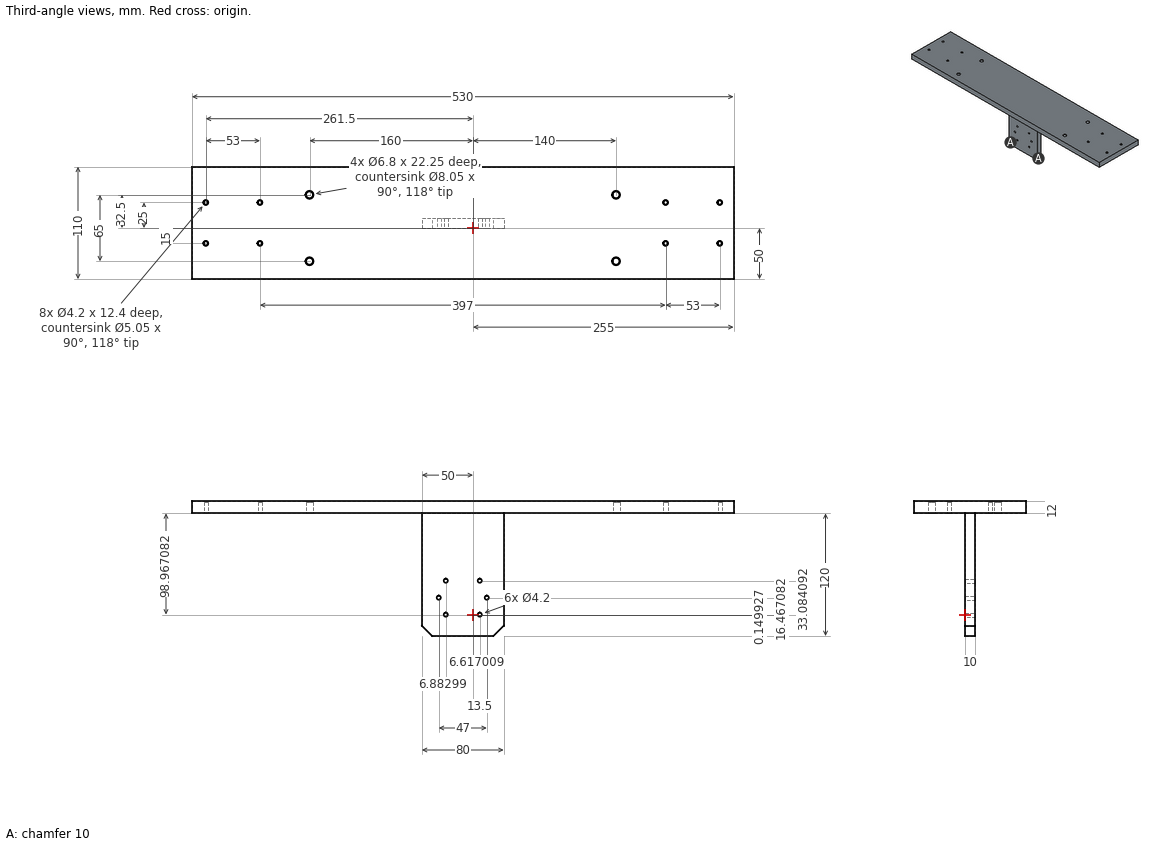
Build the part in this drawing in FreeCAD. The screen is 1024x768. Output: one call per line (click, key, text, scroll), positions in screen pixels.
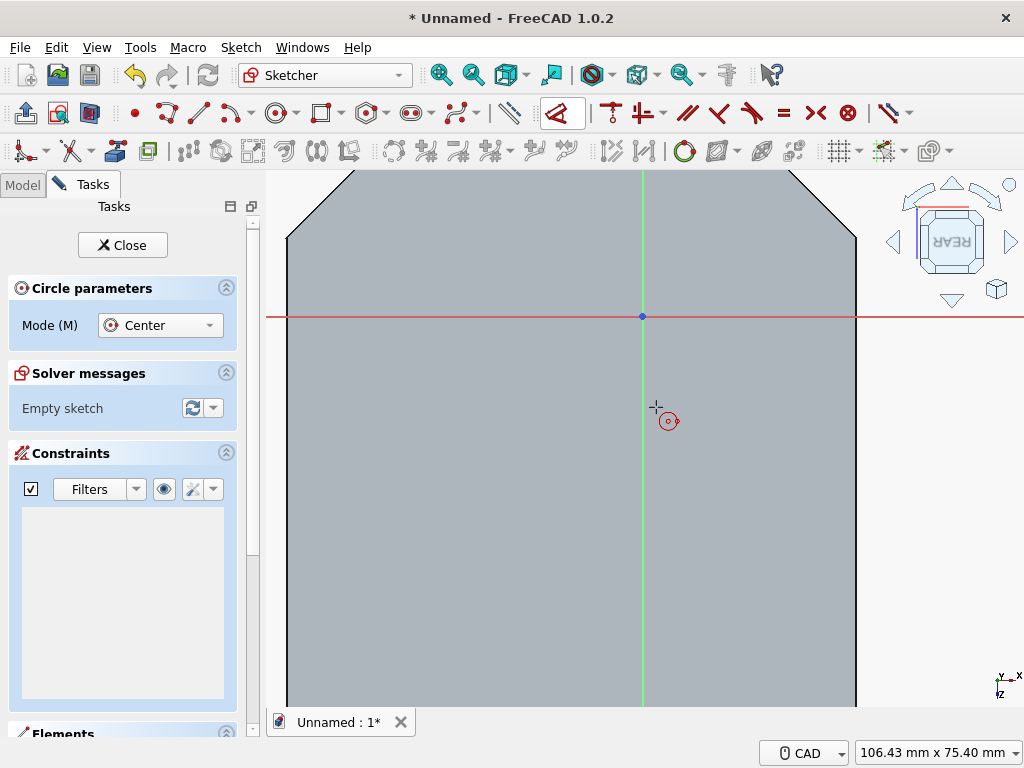
scroll(690, 316, up, 14)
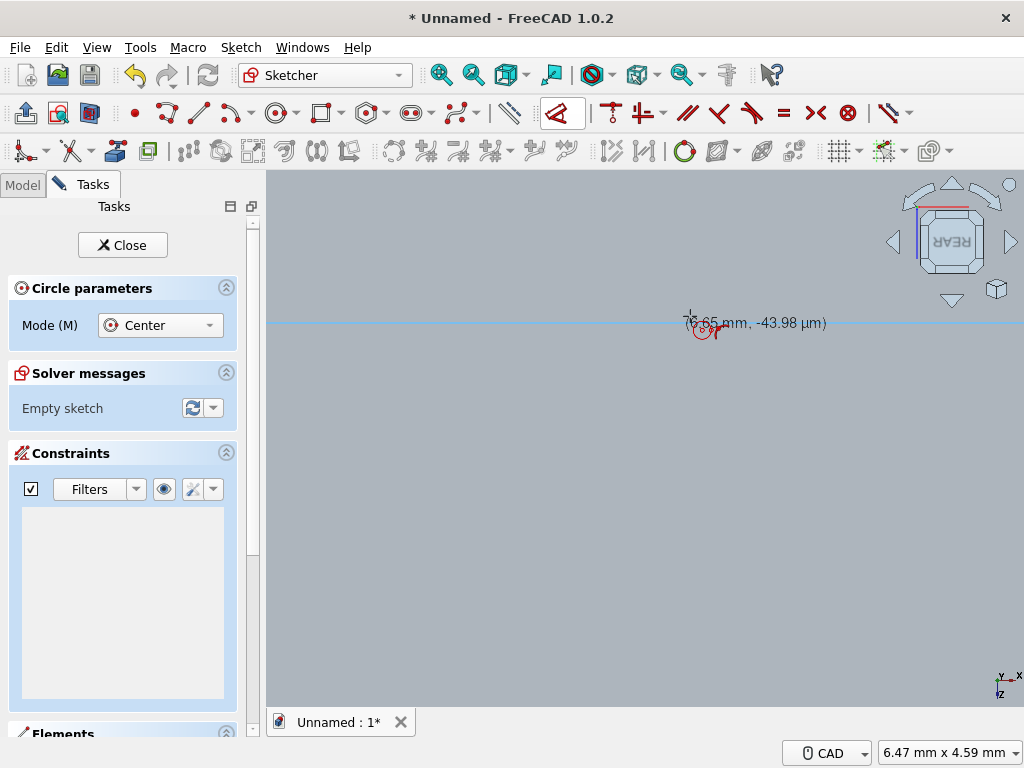
click(678, 306)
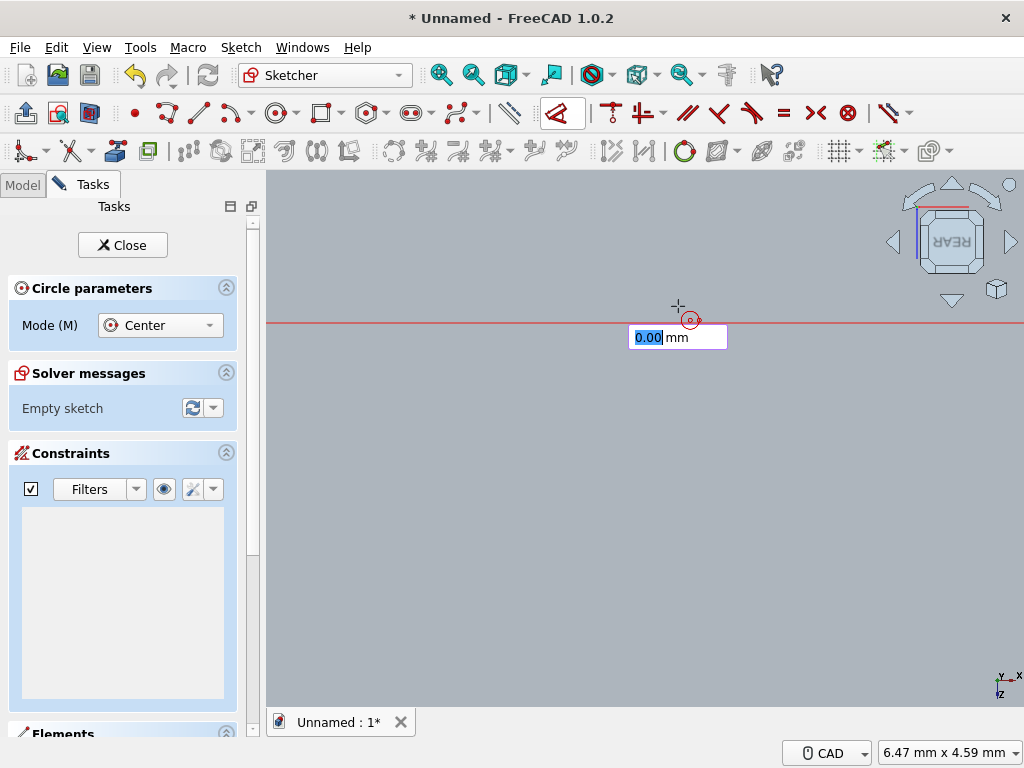
scroll(696, 321, down, 14)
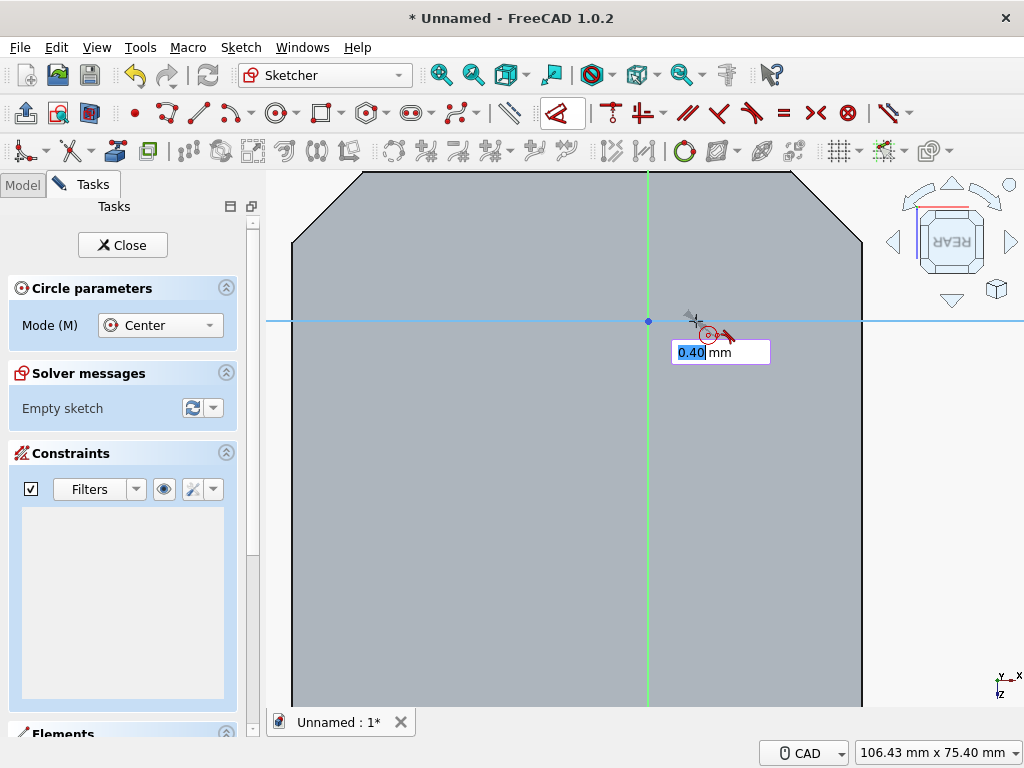
scroll(706, 310, up, 2)
move(706, 309)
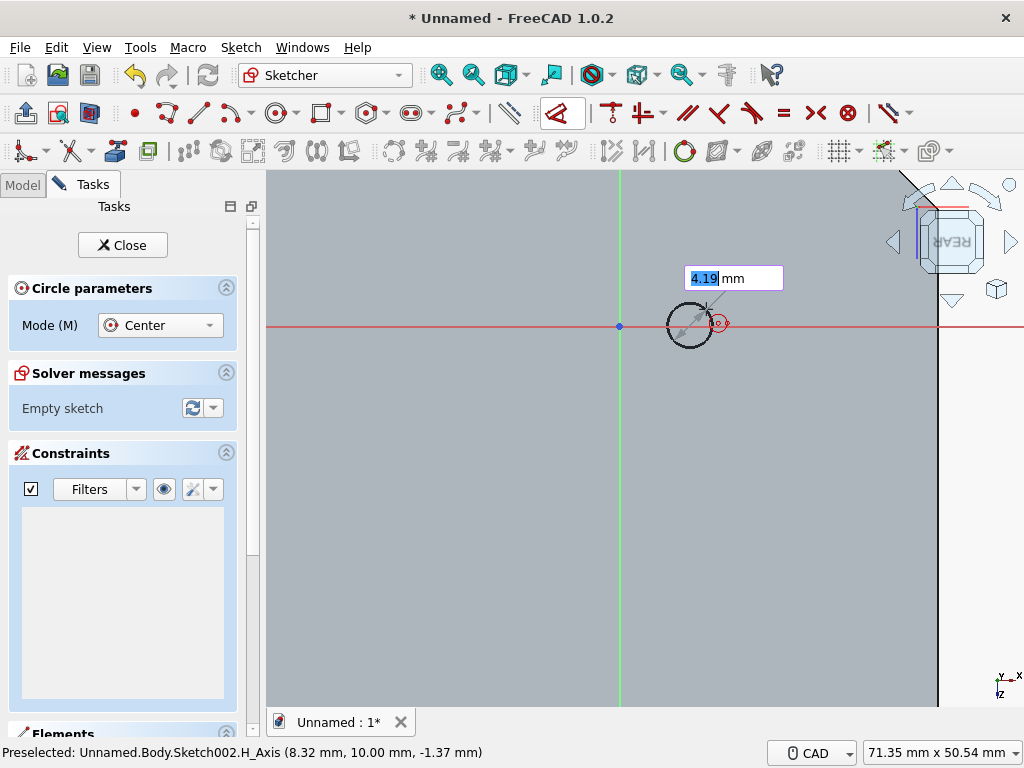
text(4.2)
key(Return)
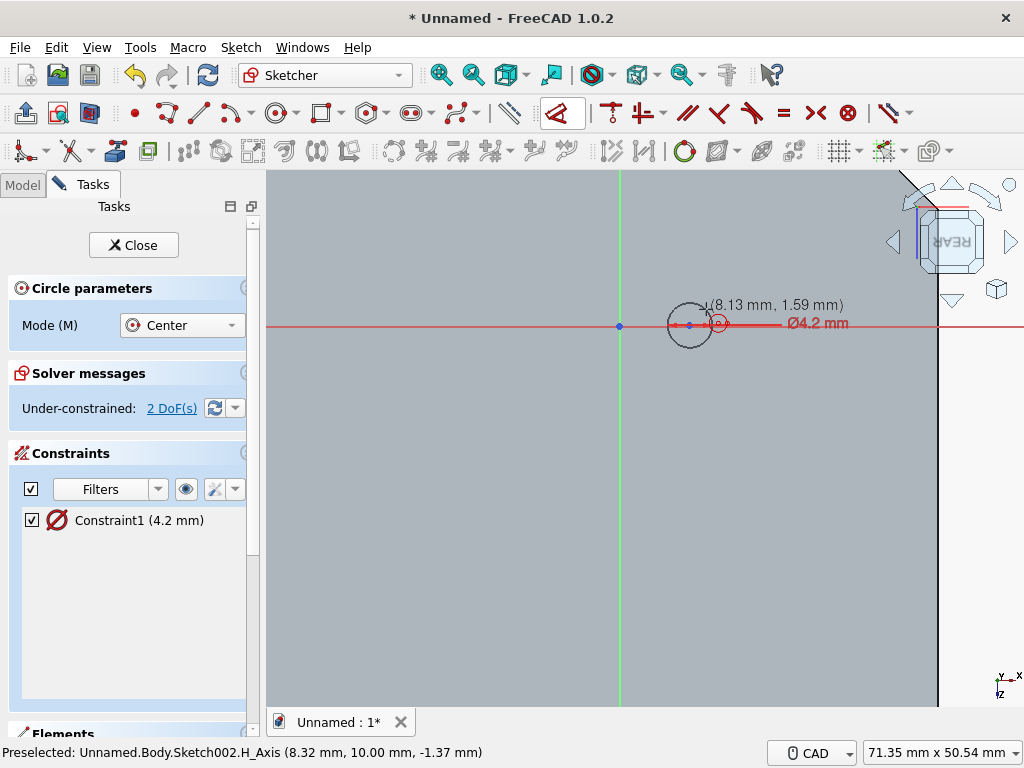
click(763, 502)
move(779, 486)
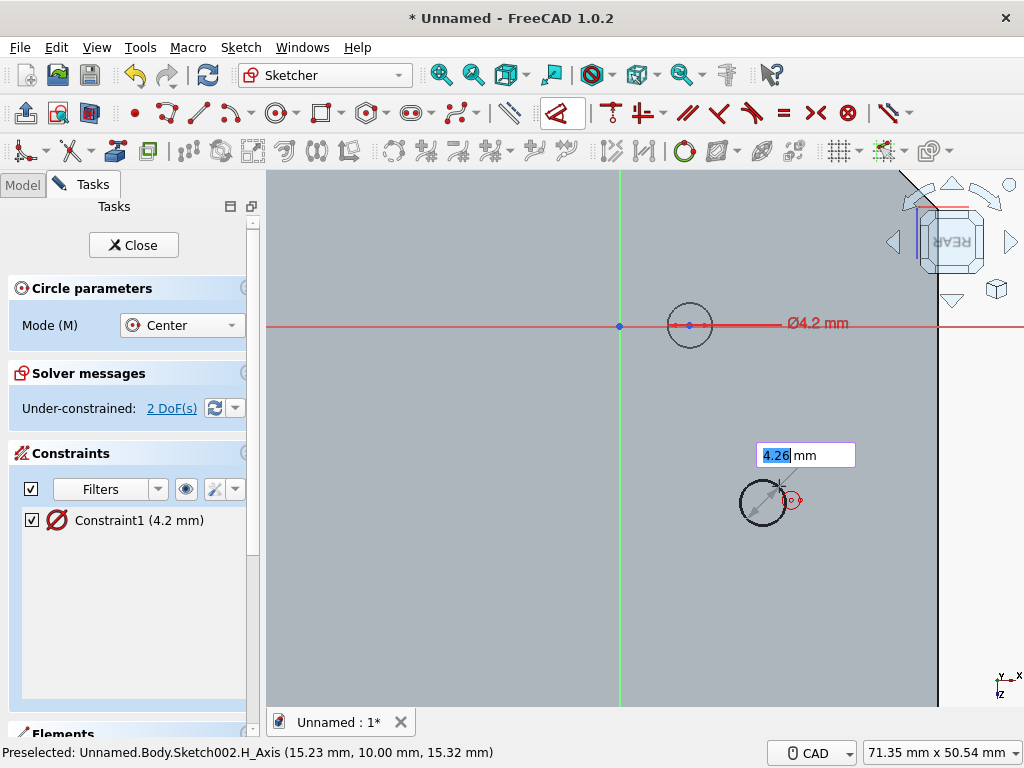
text(4.2)
key(Return)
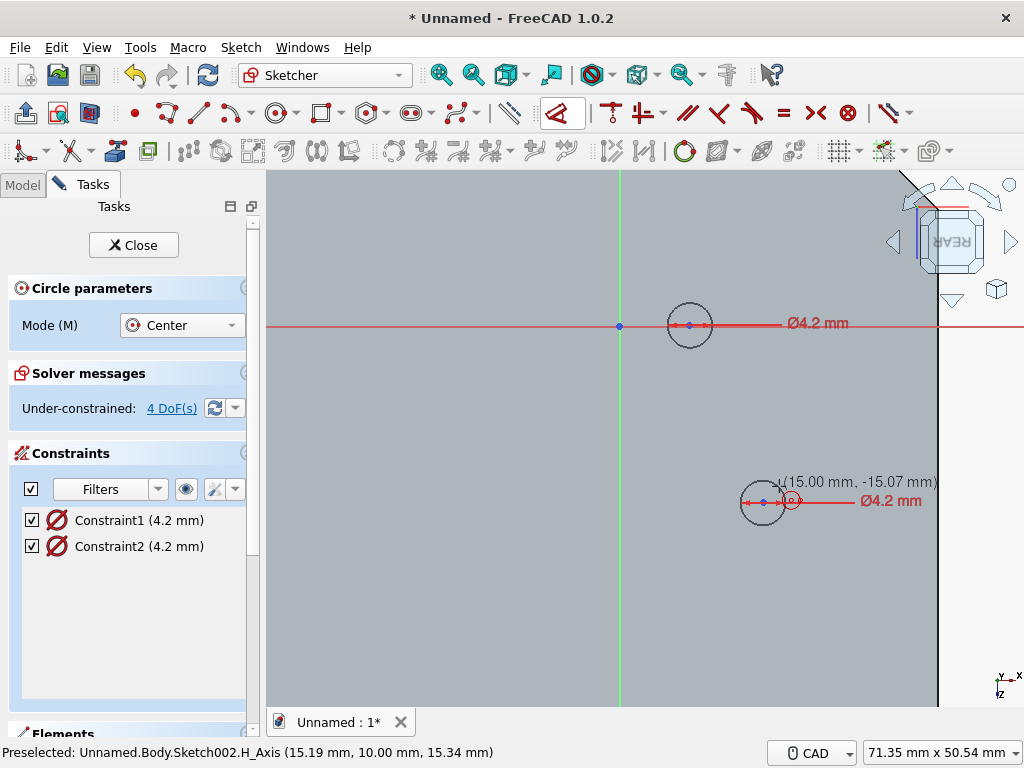
click(690, 678)
move(706, 663)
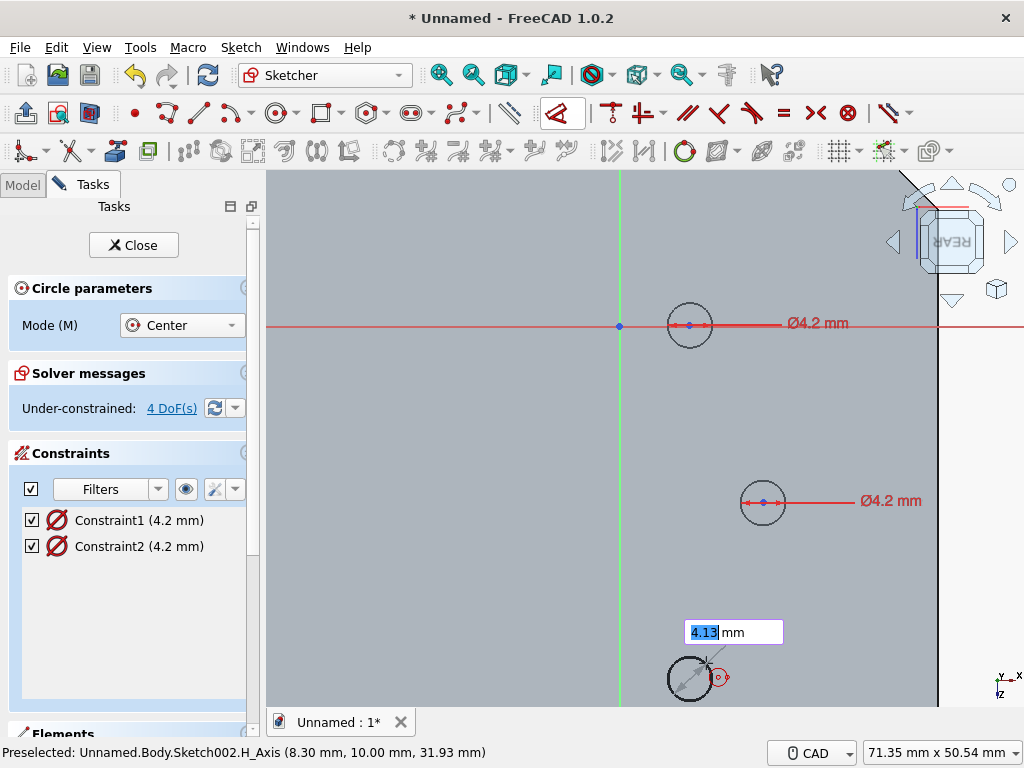
text(4.2)
key(Return)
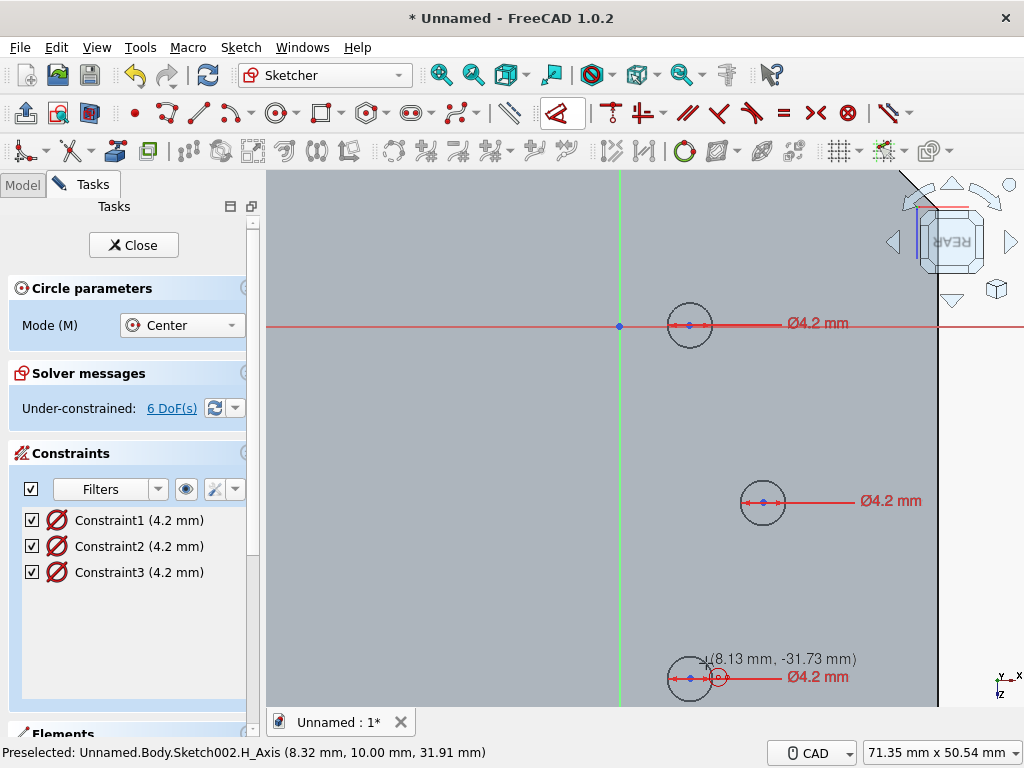
click(337, 678)
move(353, 663)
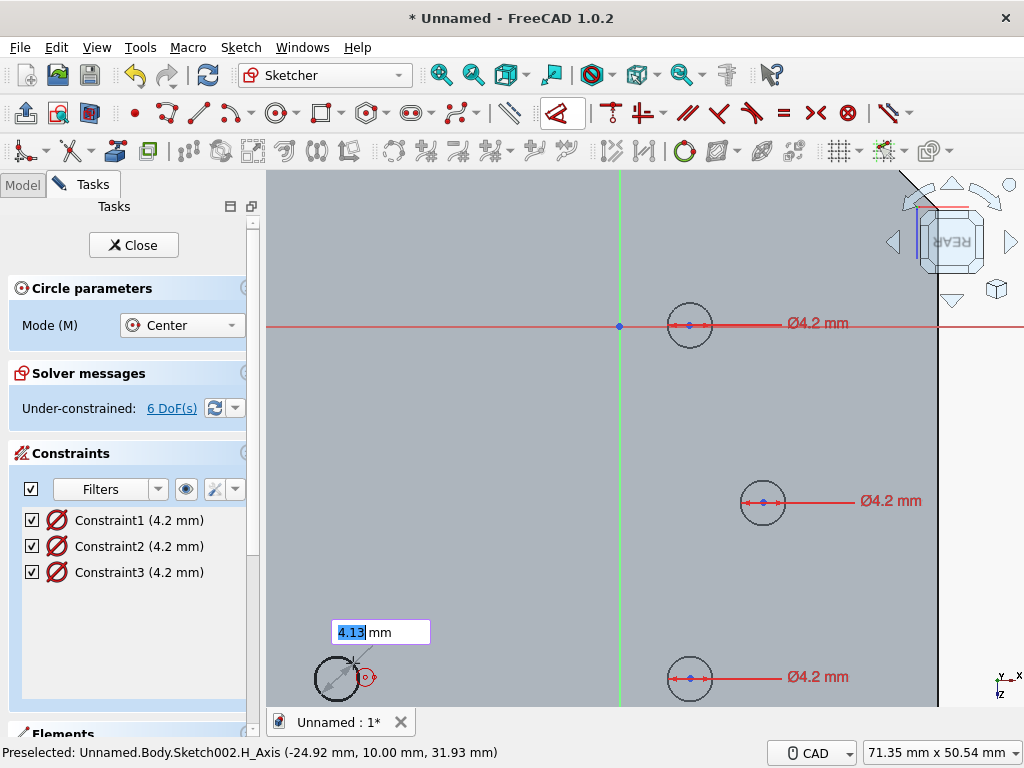
text(4.2)
key(Return)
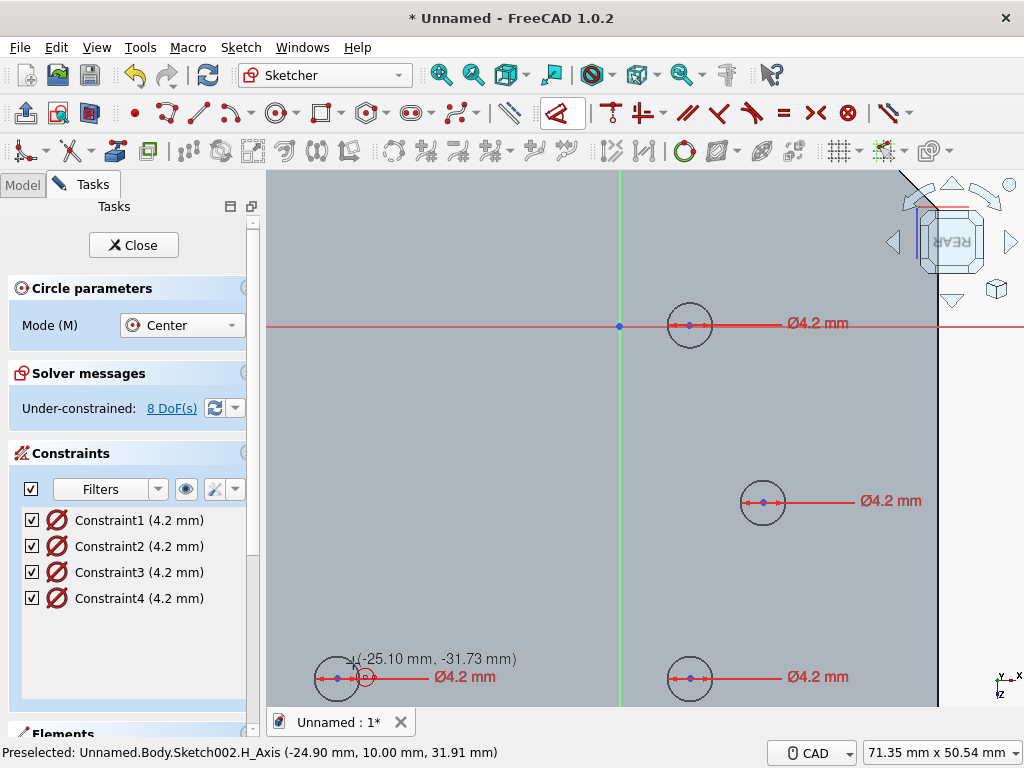
scroll(705, 310, down, 2)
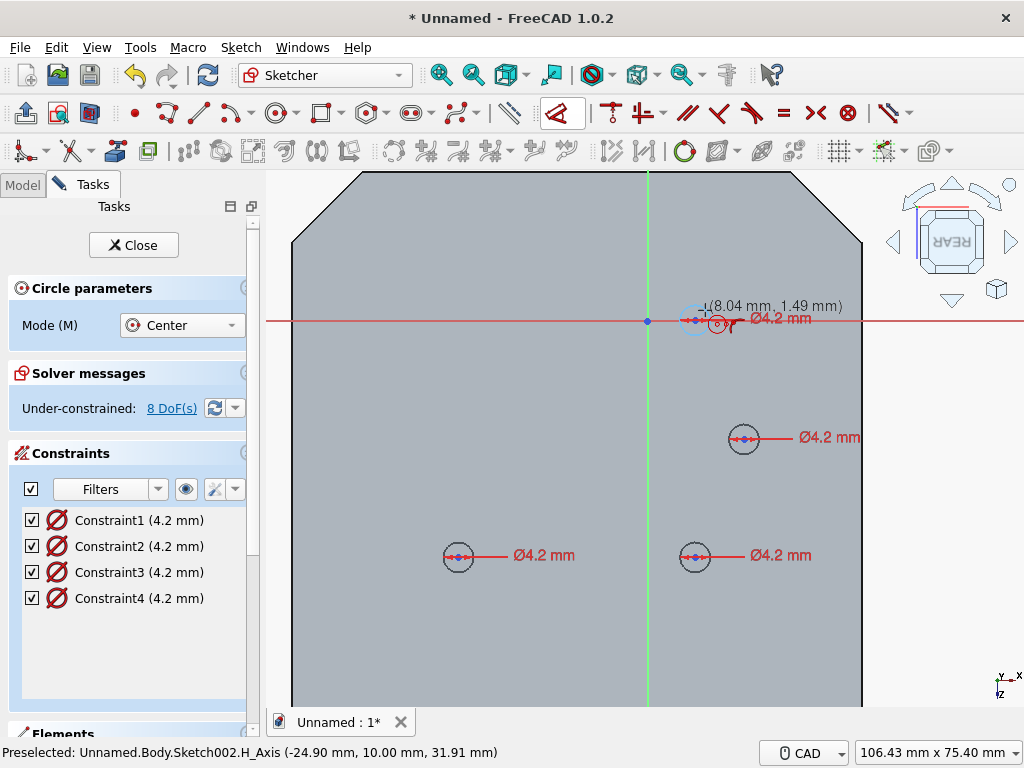
scroll(409, 439, up, 3)